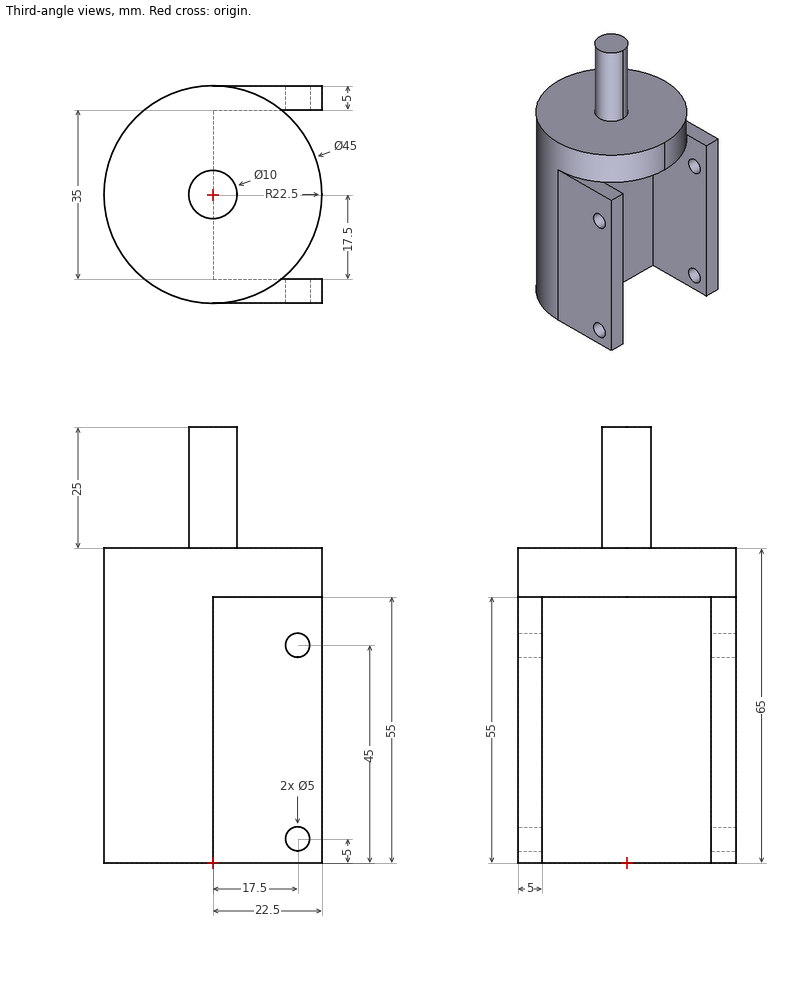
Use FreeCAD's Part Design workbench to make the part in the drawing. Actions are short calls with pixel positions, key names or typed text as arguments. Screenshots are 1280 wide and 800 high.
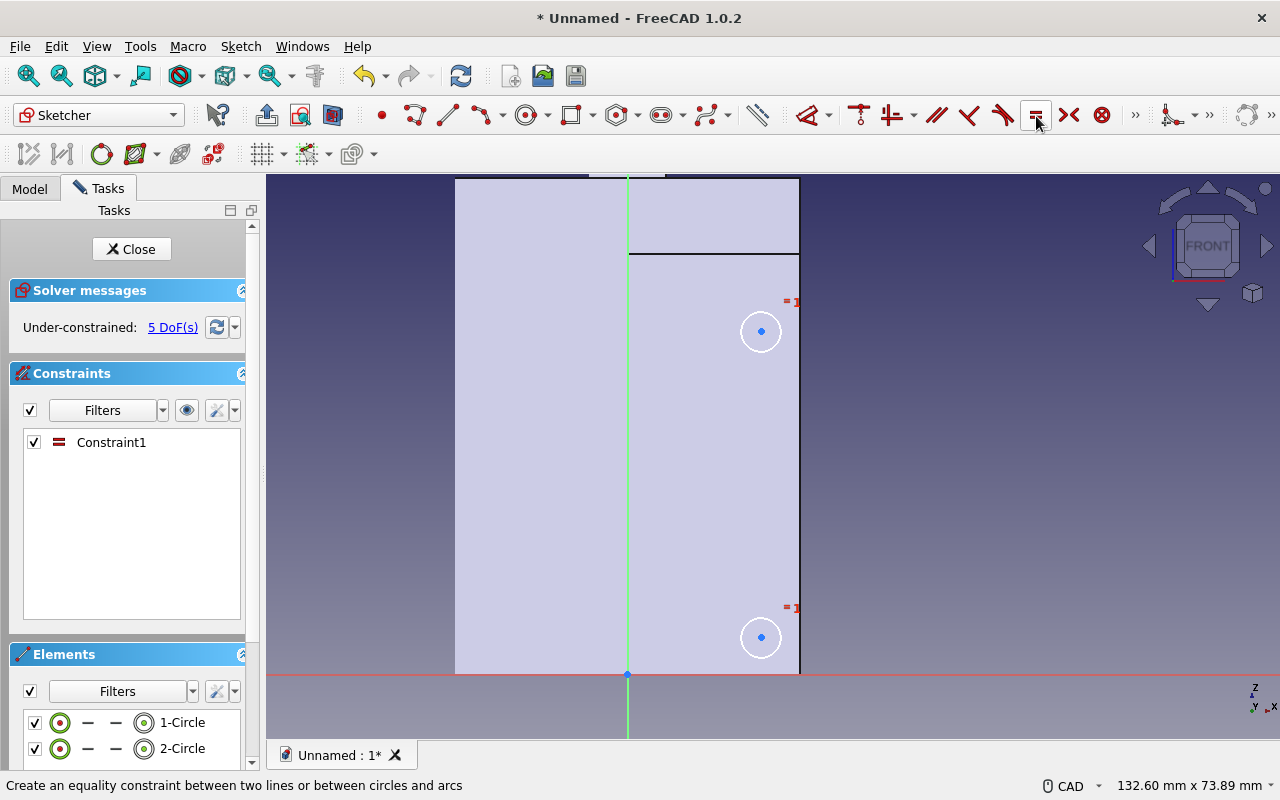
click(806, 116)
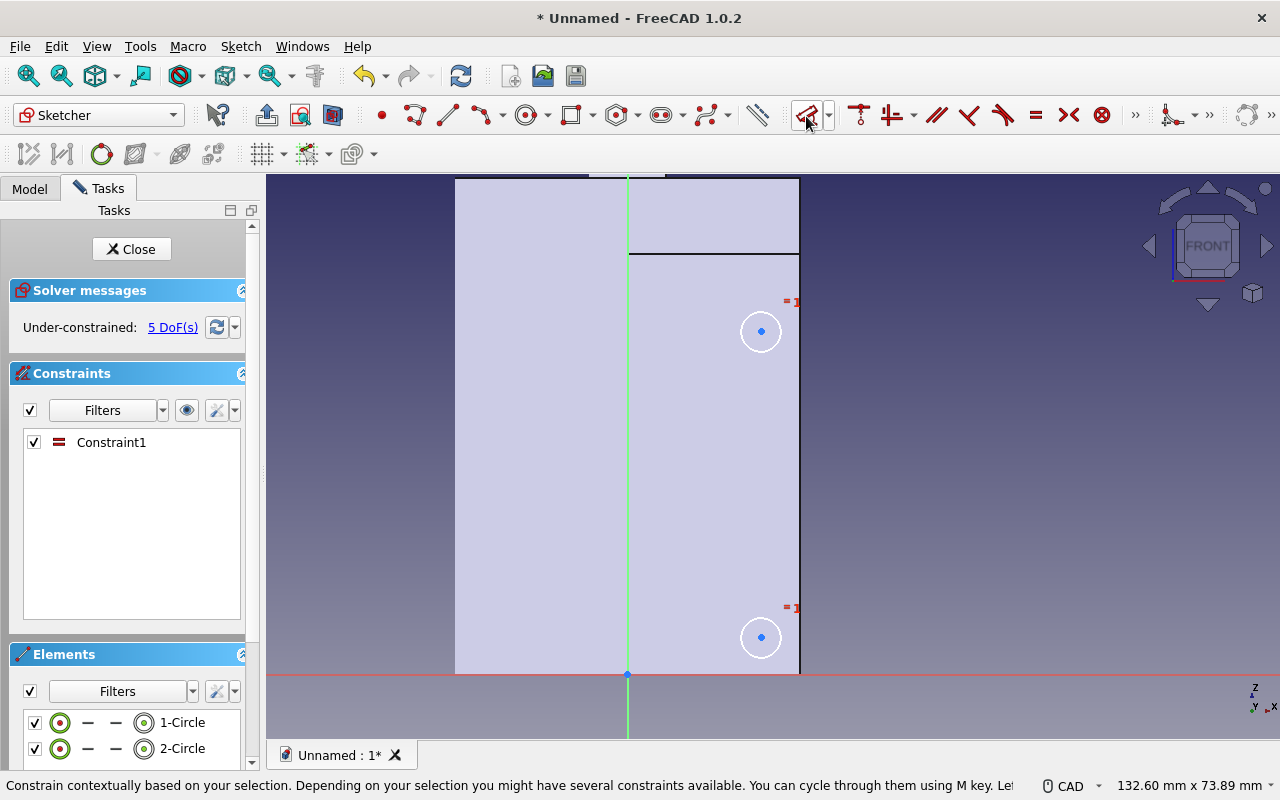
click(775, 624)
click(798, 601)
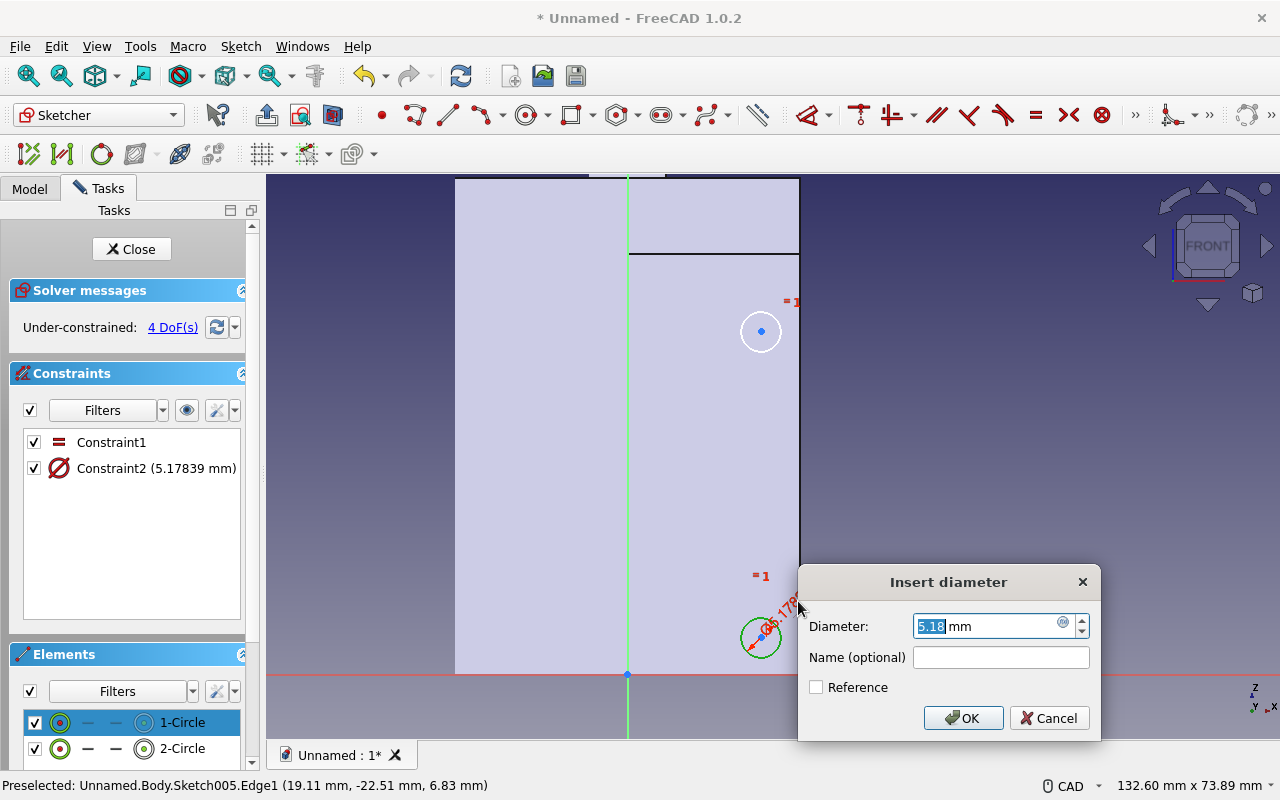
text(5)
key(Return)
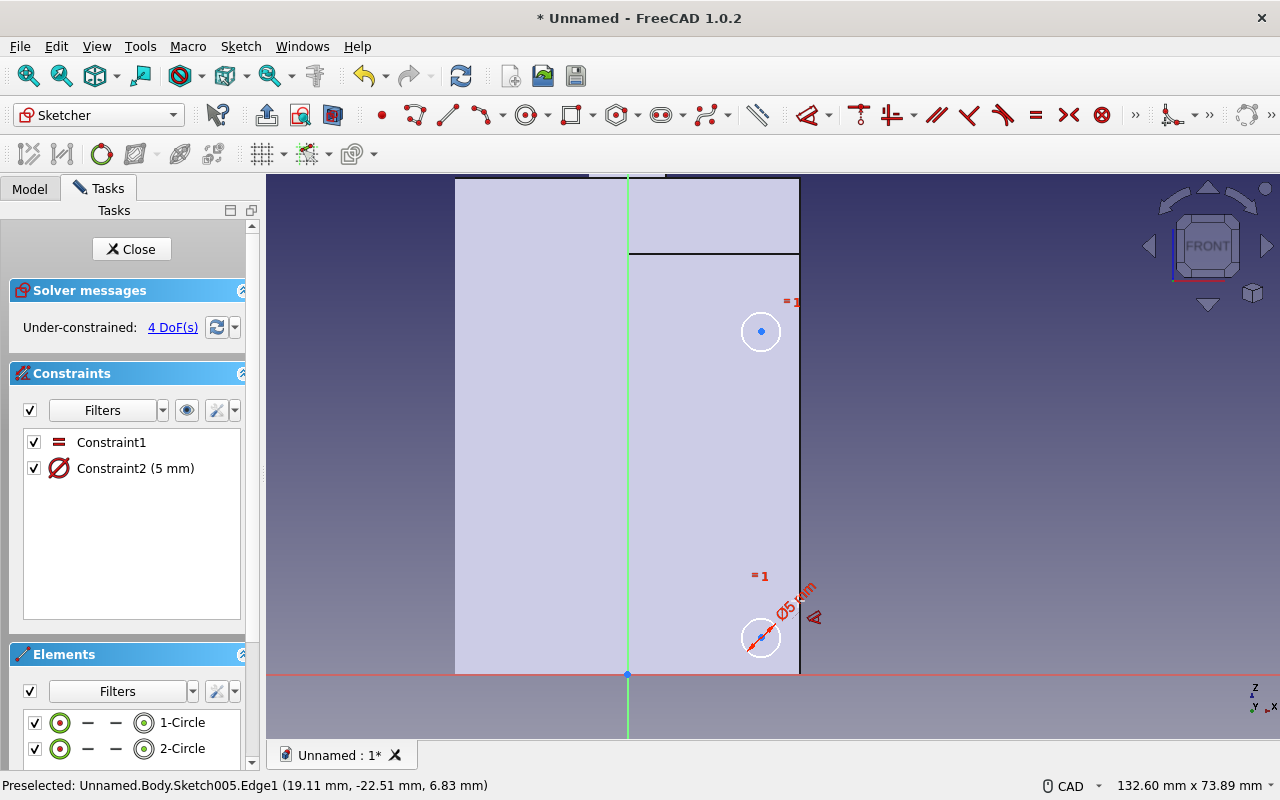
click(761, 638)
click(594, 656)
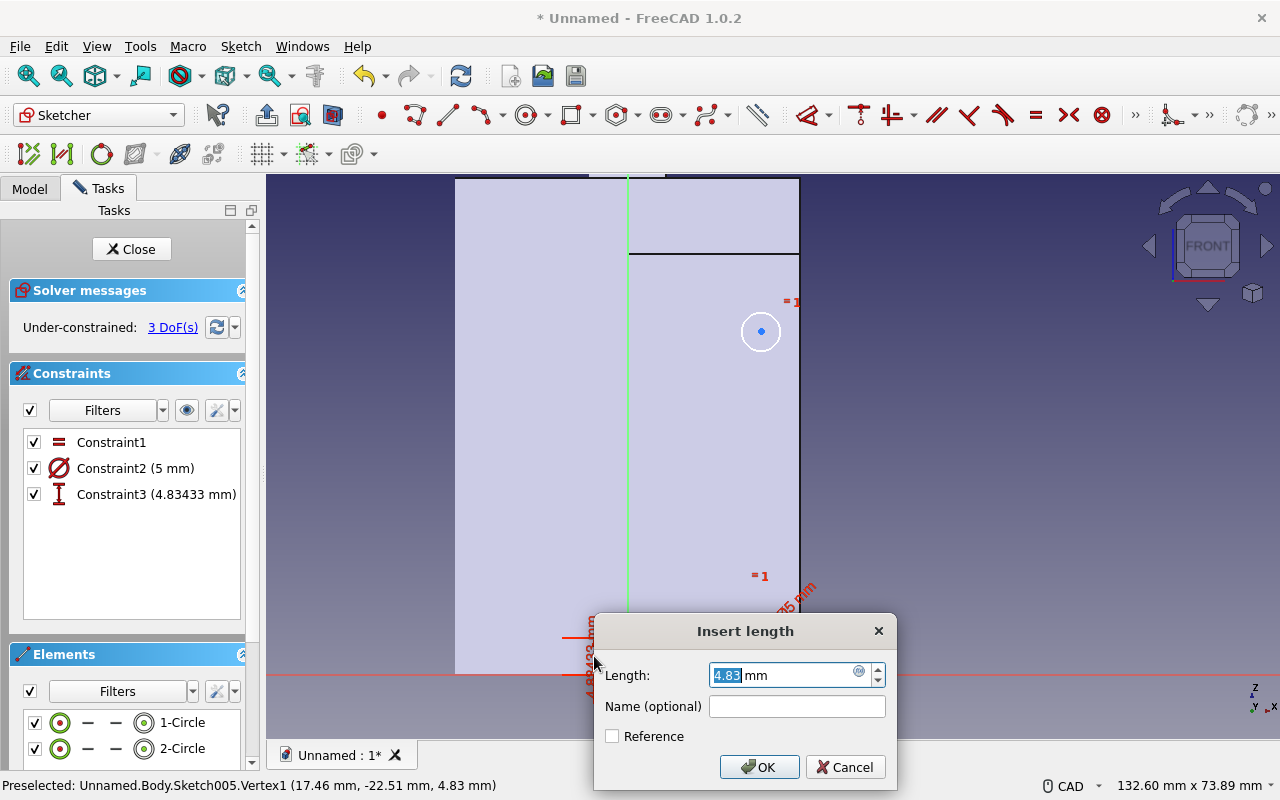
text(5)
key(Return)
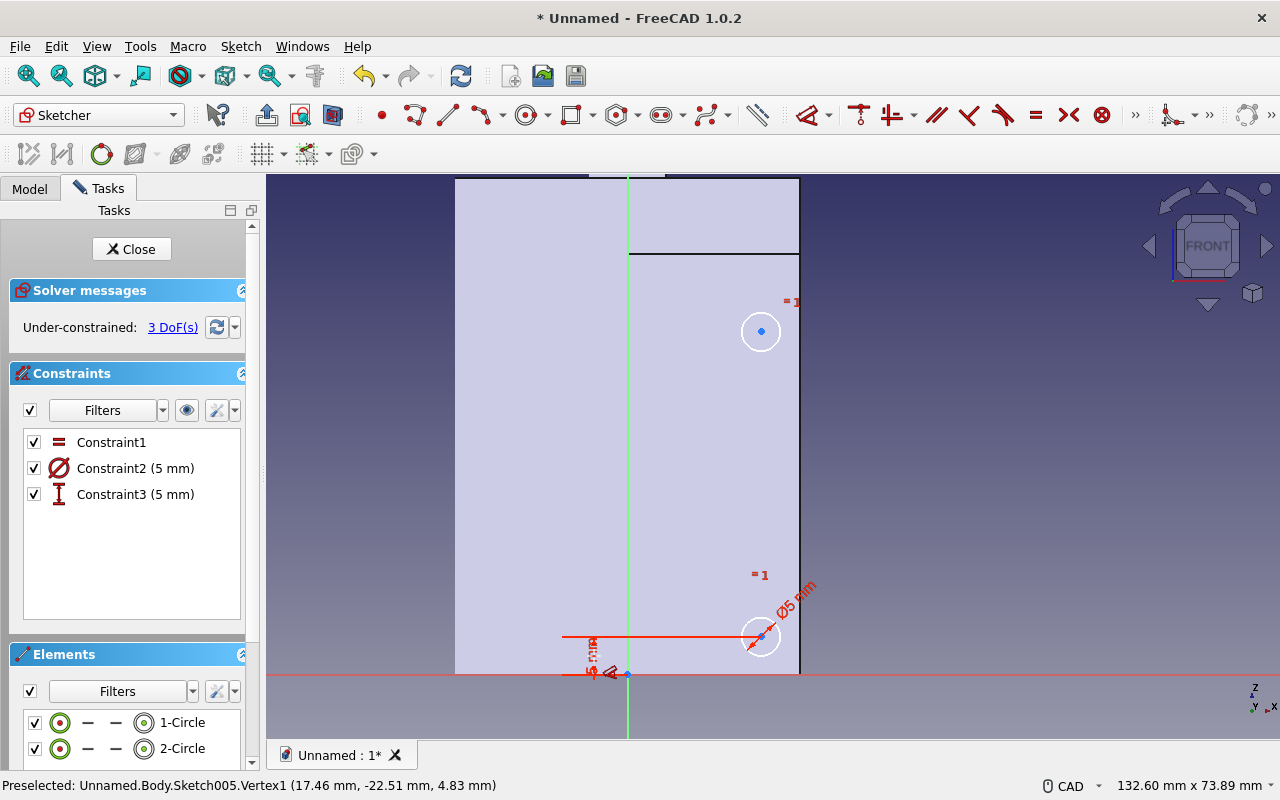
click(761, 332)
click(594, 503)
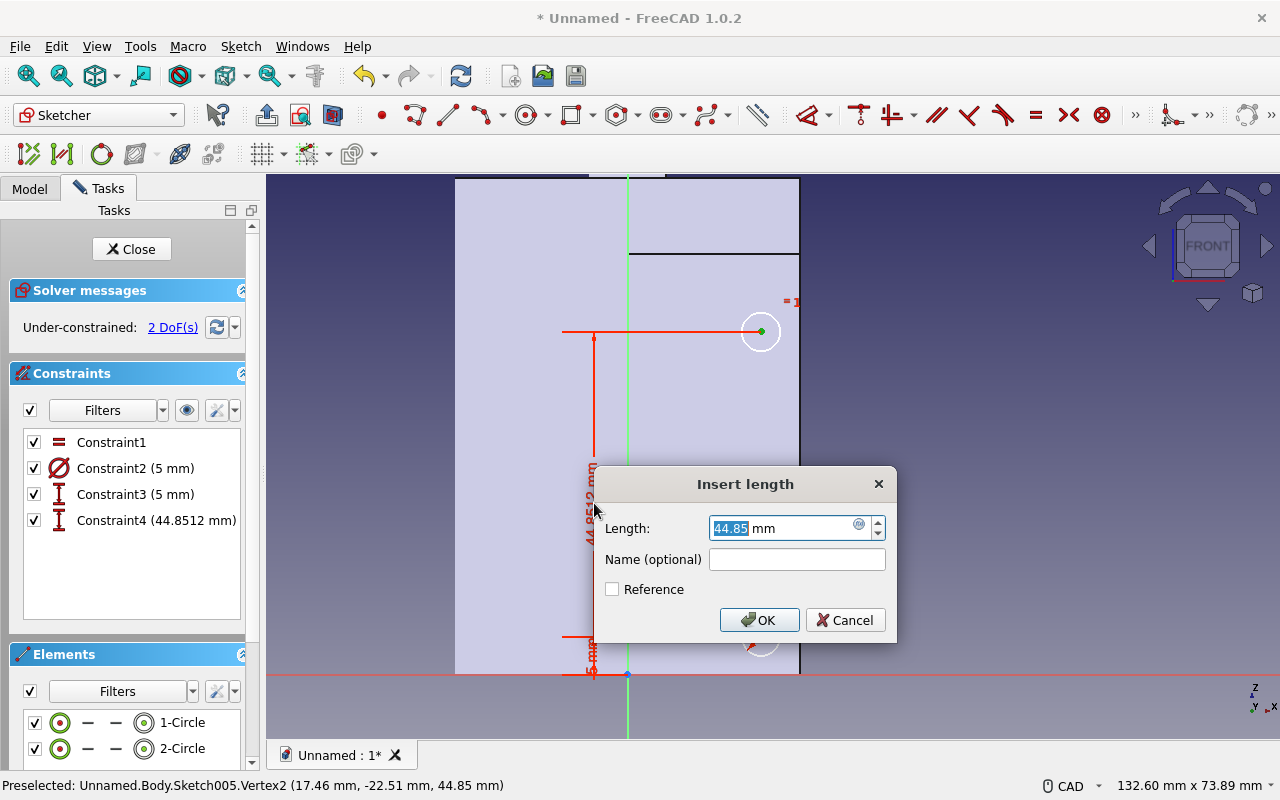
text(45)
key(Return)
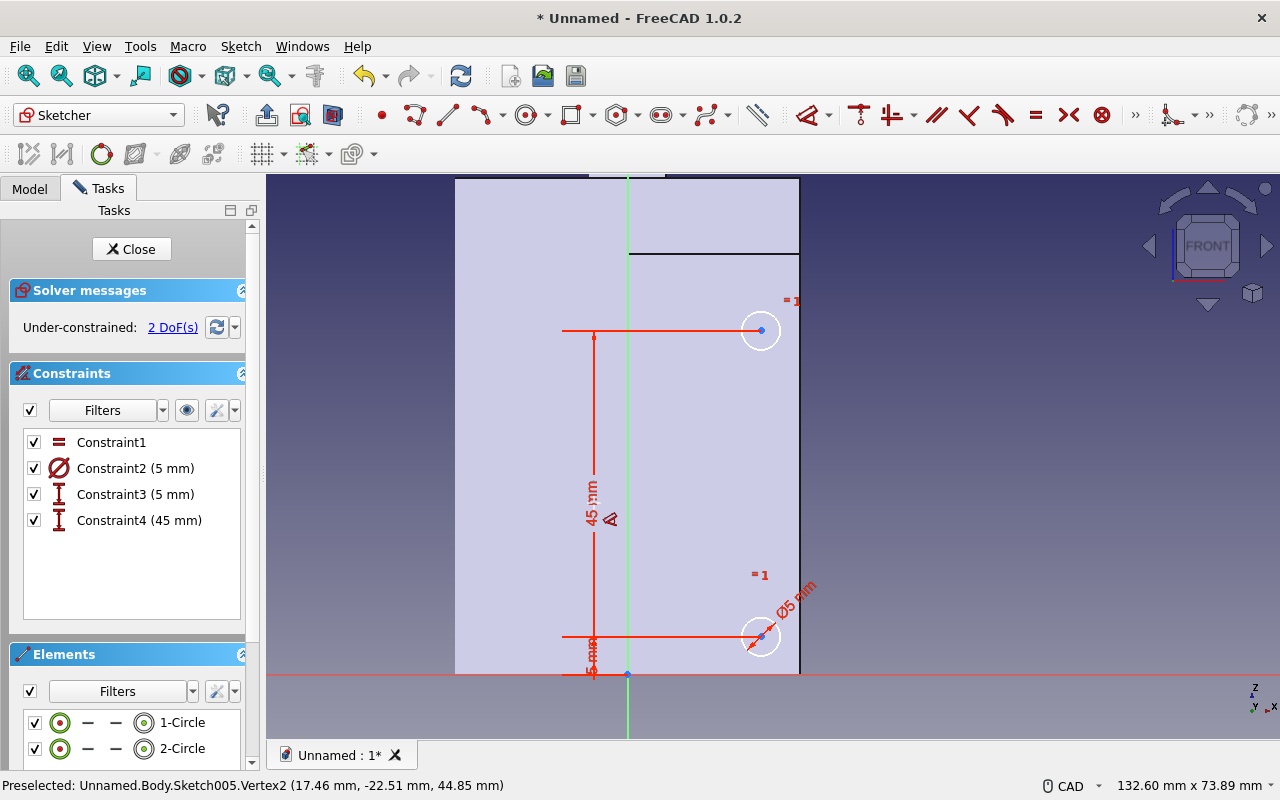
click(761, 637)
click(694, 709)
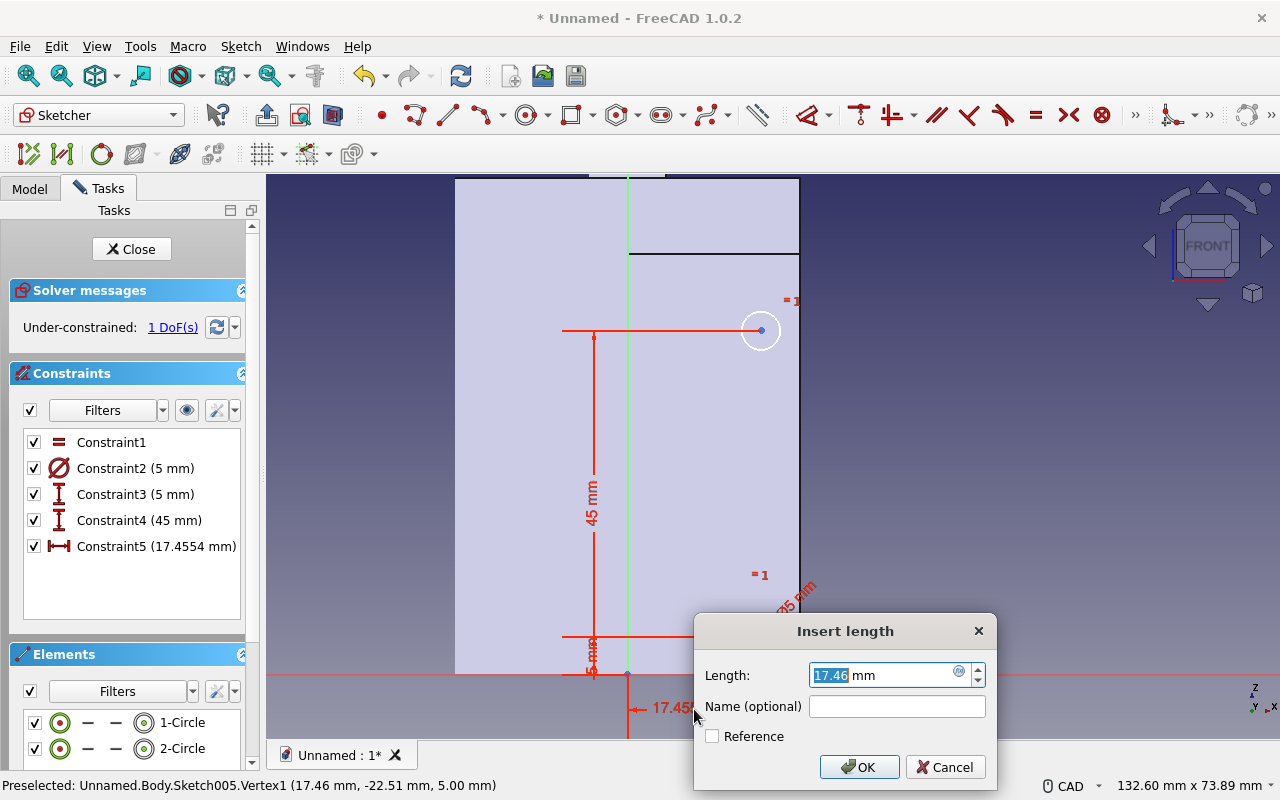
text(17.5)
key(Return)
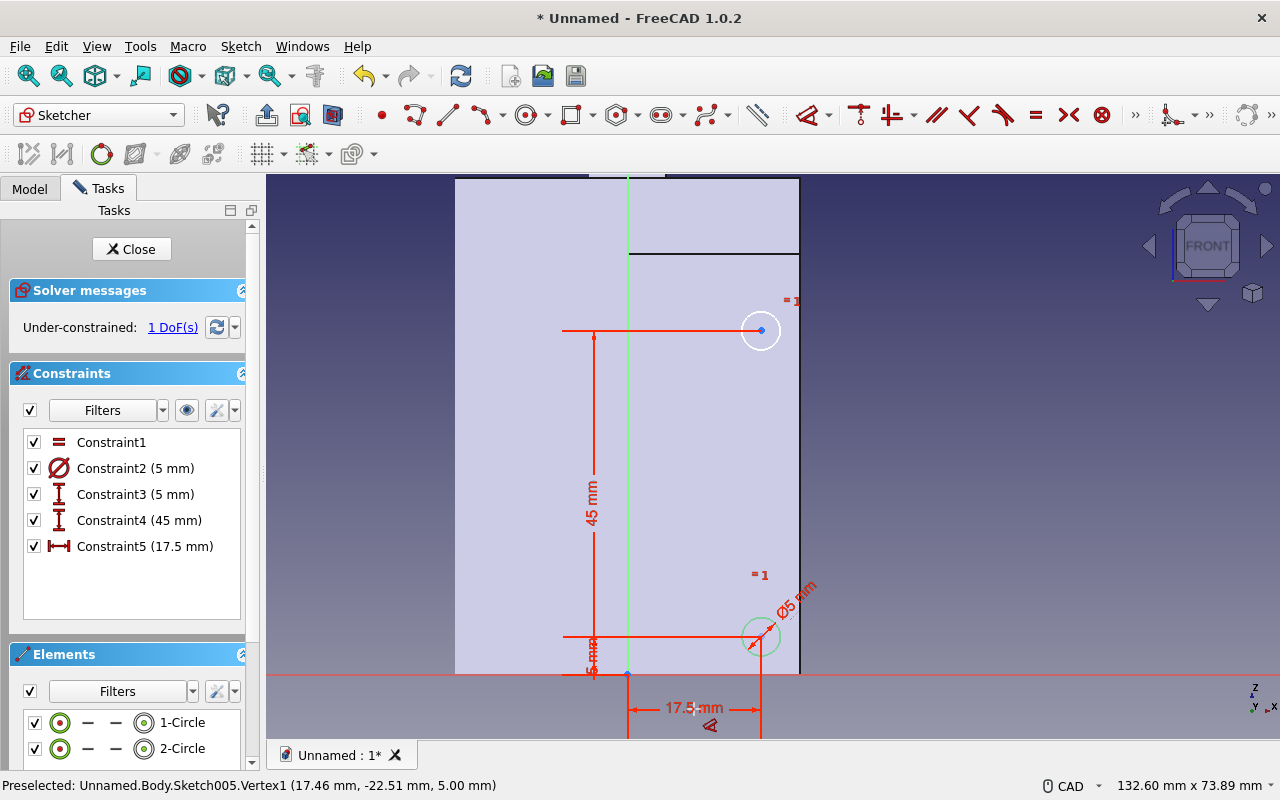
click(761, 331)
click(694, 297)